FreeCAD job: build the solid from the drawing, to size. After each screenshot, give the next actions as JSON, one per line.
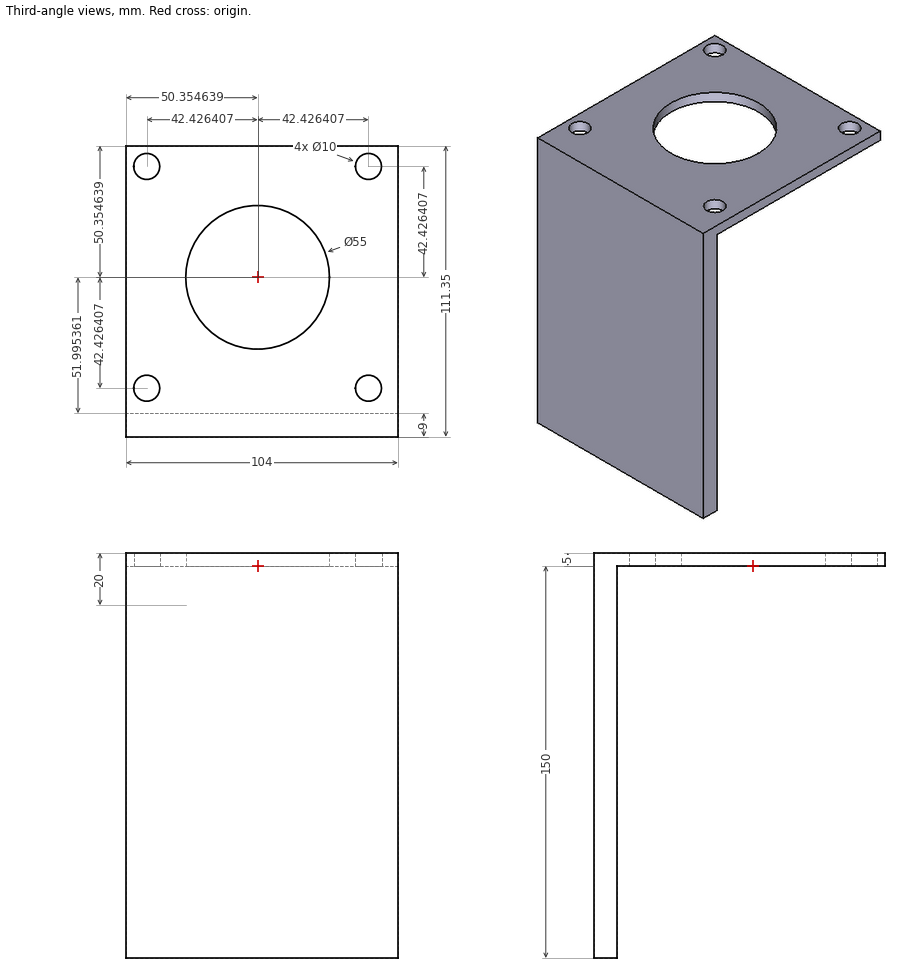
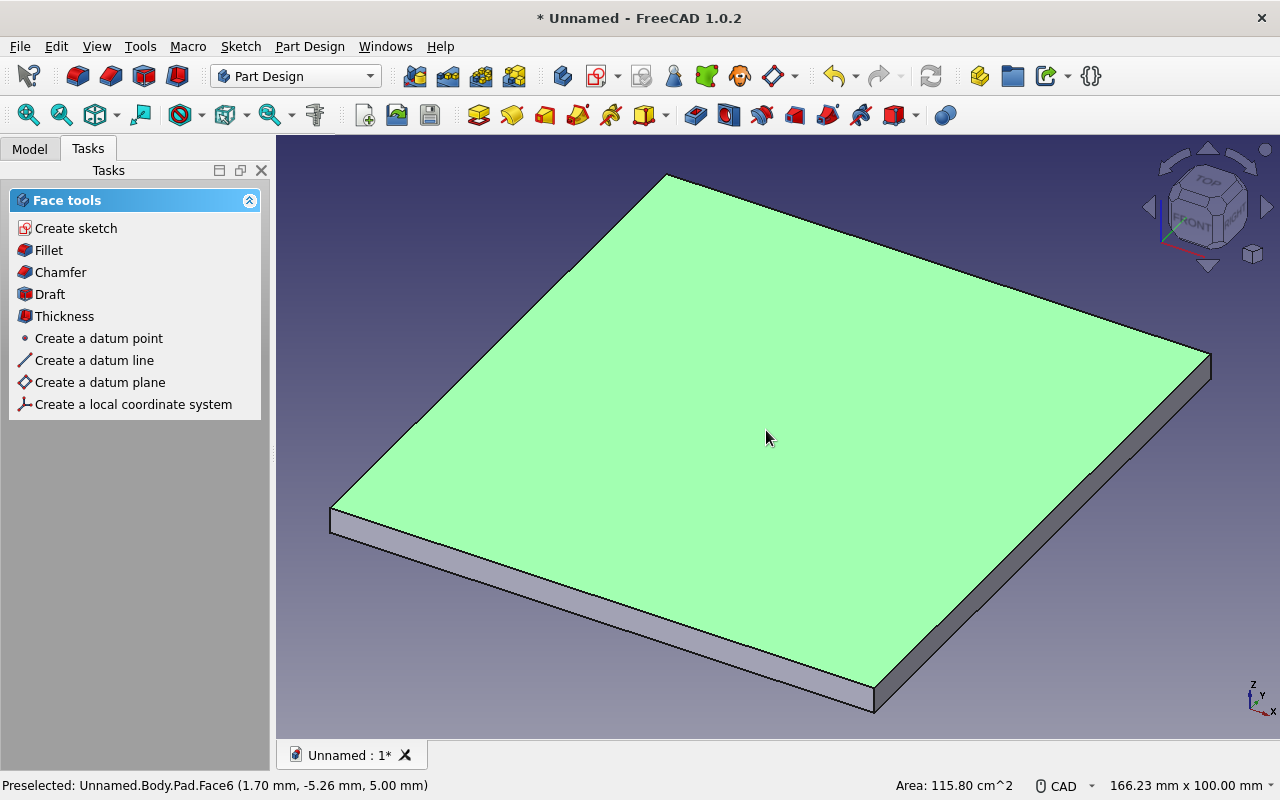
{"action": "left_click", "coordinate": [596, 76]}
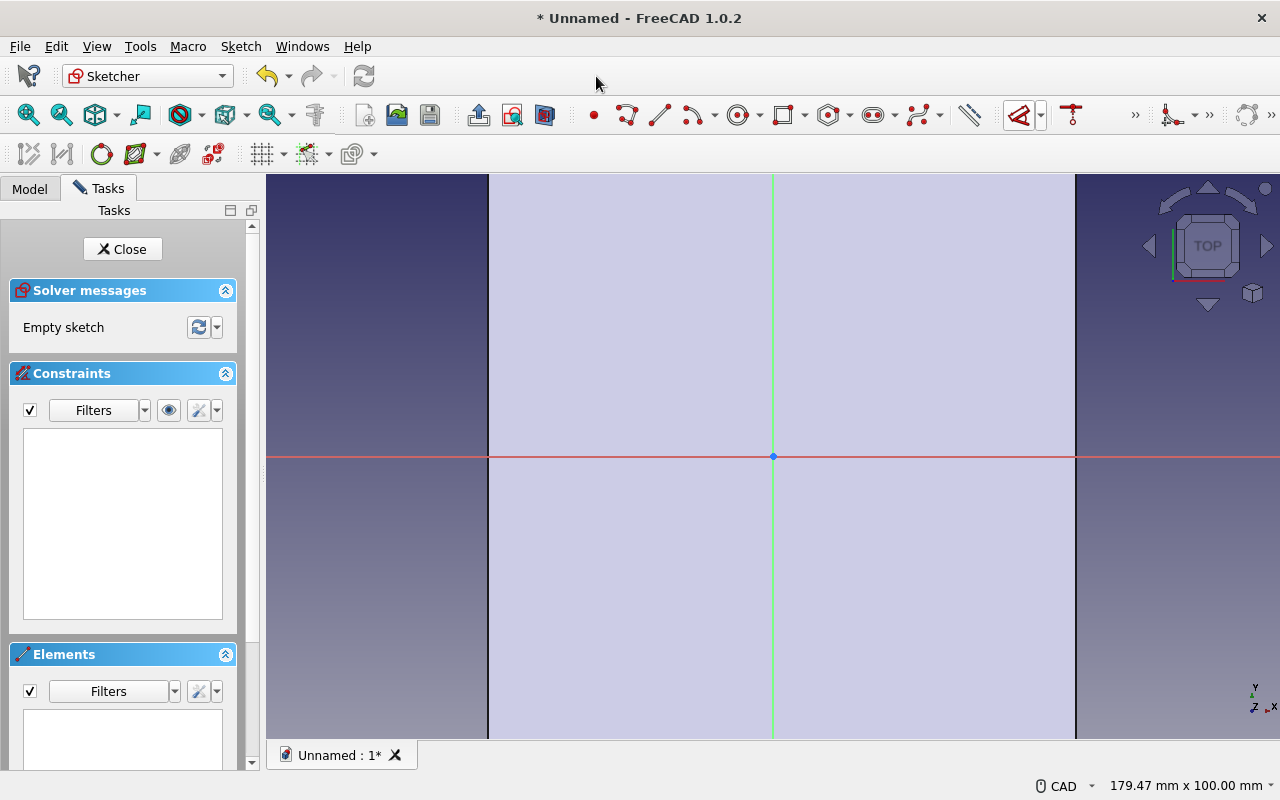
{"action": "key", "text": "g c"}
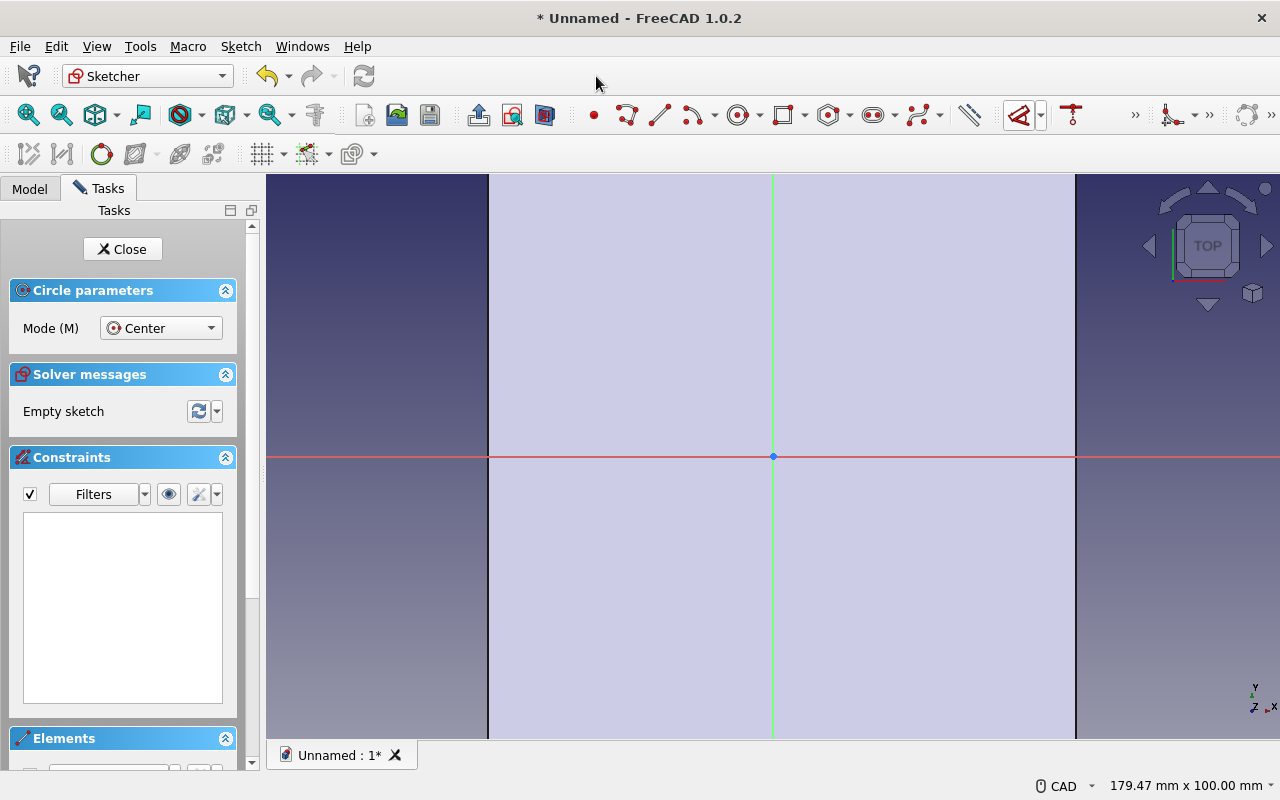
{"action": "left_click", "coordinate": [773, 456]}
{"action": "mouse_move", "coordinate": [883, 347]}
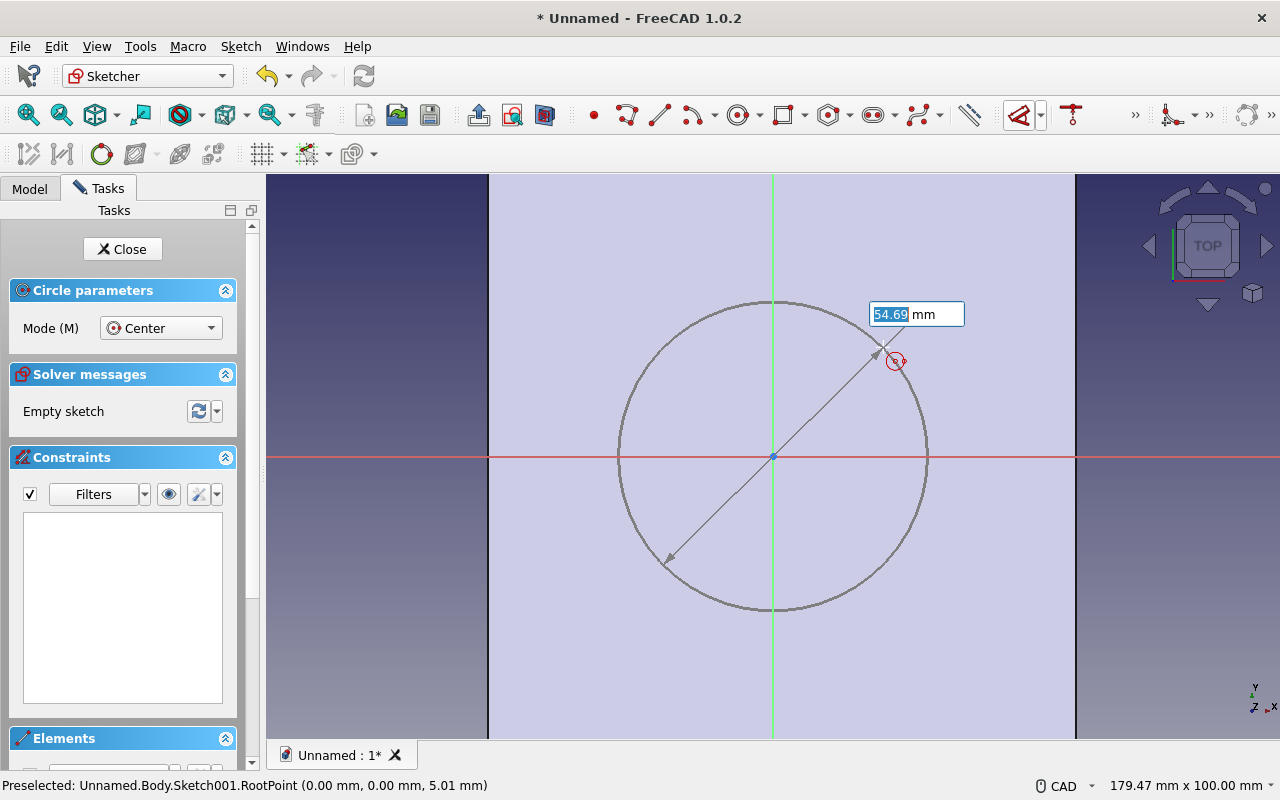
{"action": "type", "text": "55"}
{"action": "key", "text": "Return"}
{"action": "key", "text": "Escape"}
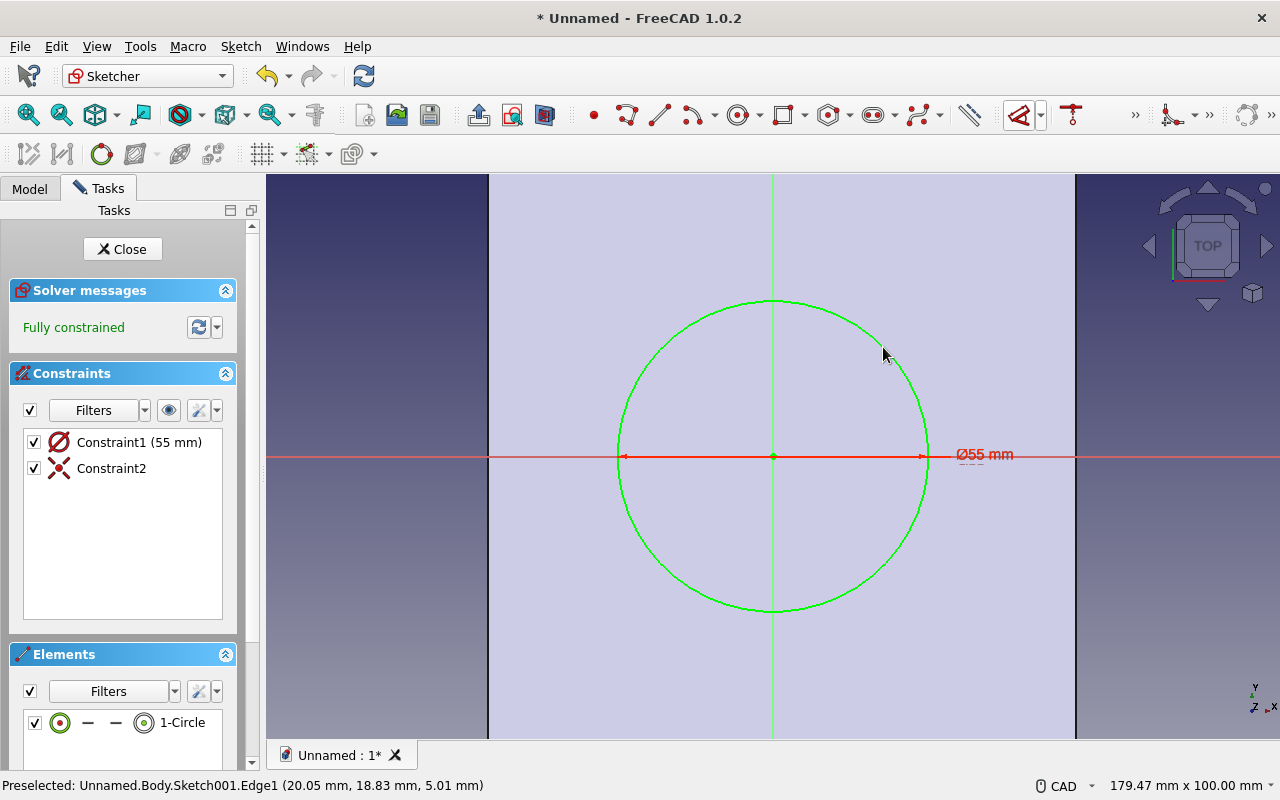
{"action": "left_click", "coordinate": [123, 249]}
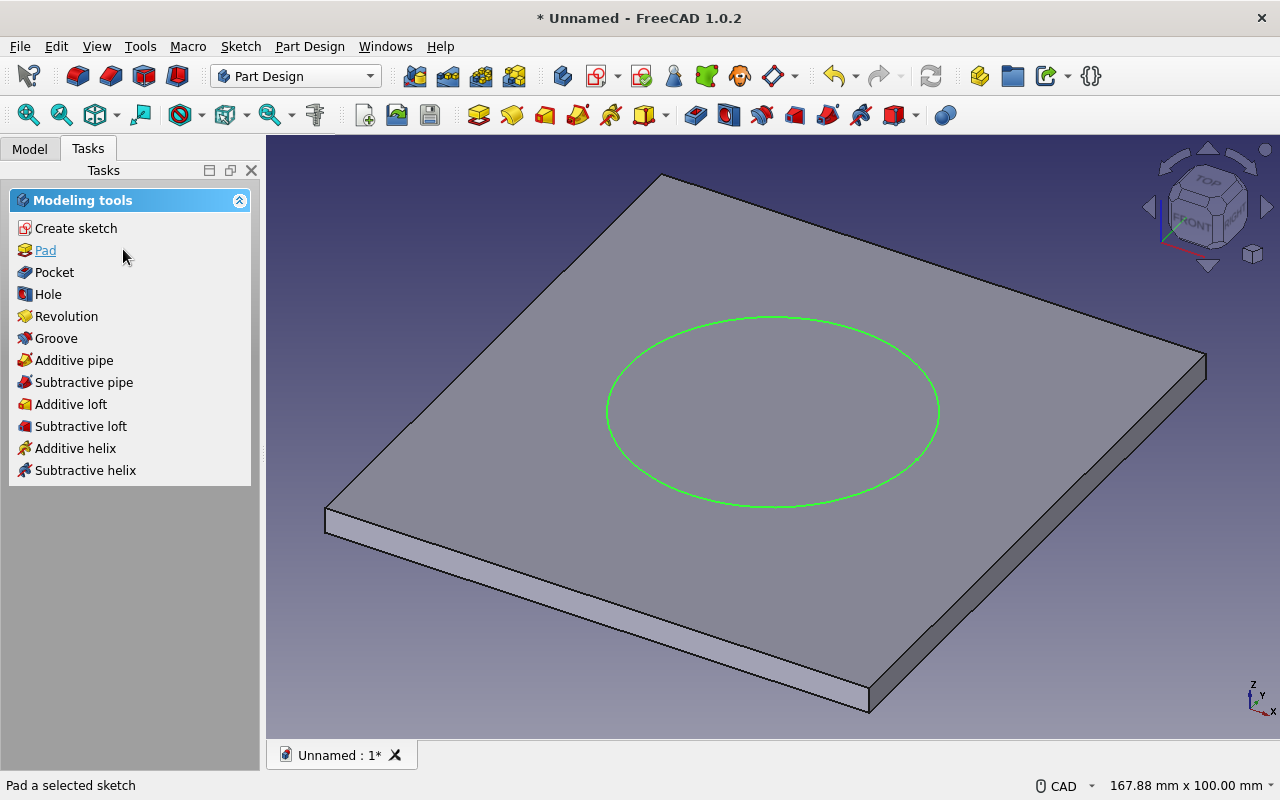
{"action": "left_click", "coordinate": [696, 116]}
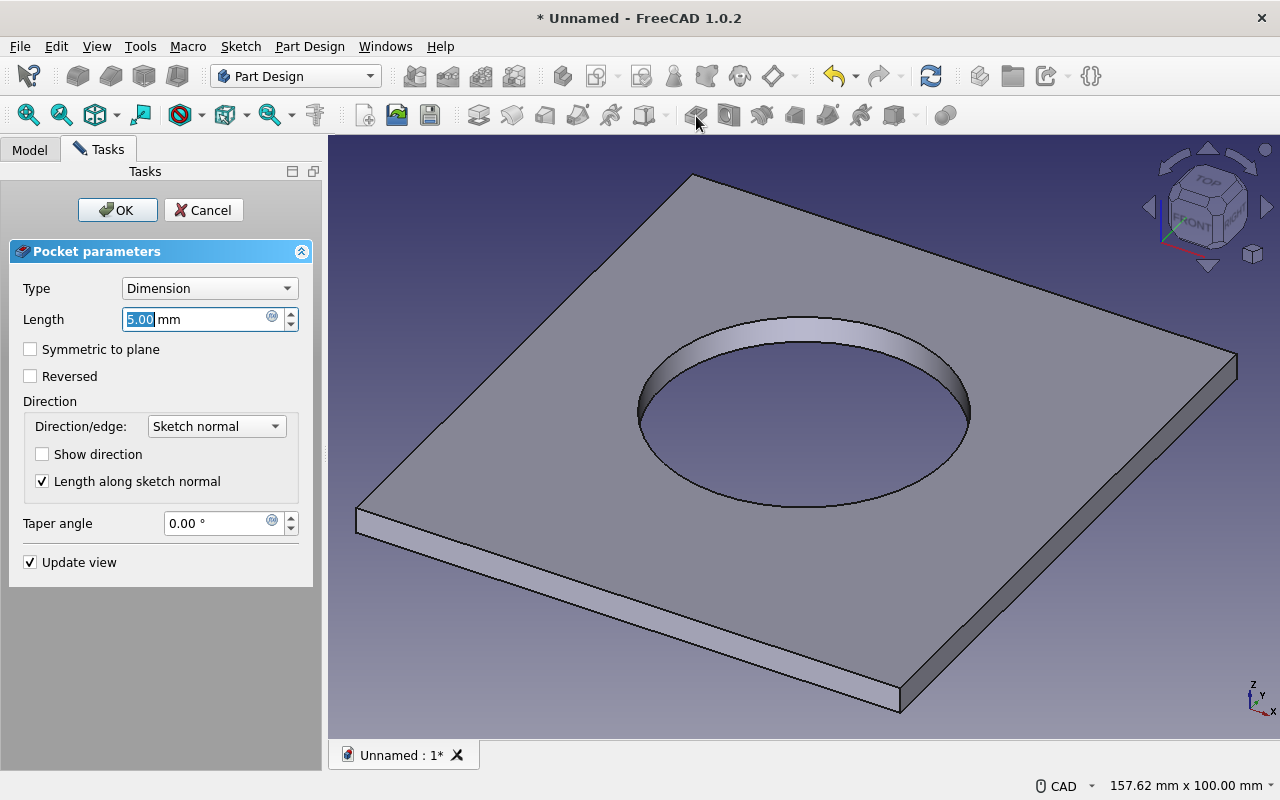
{"action": "type", "text": "20"}
{"action": "key", "text": "Tab"}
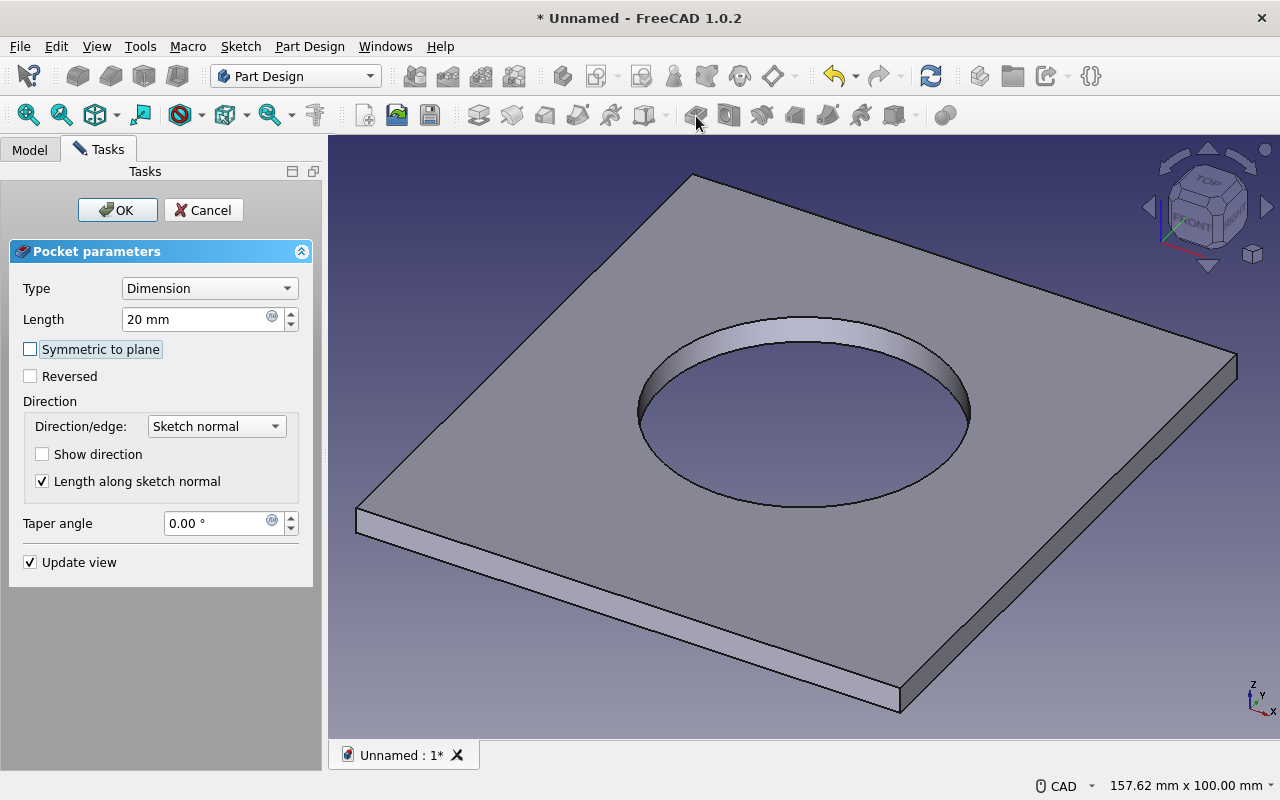
{"action": "left_click", "coordinate": [118, 210]}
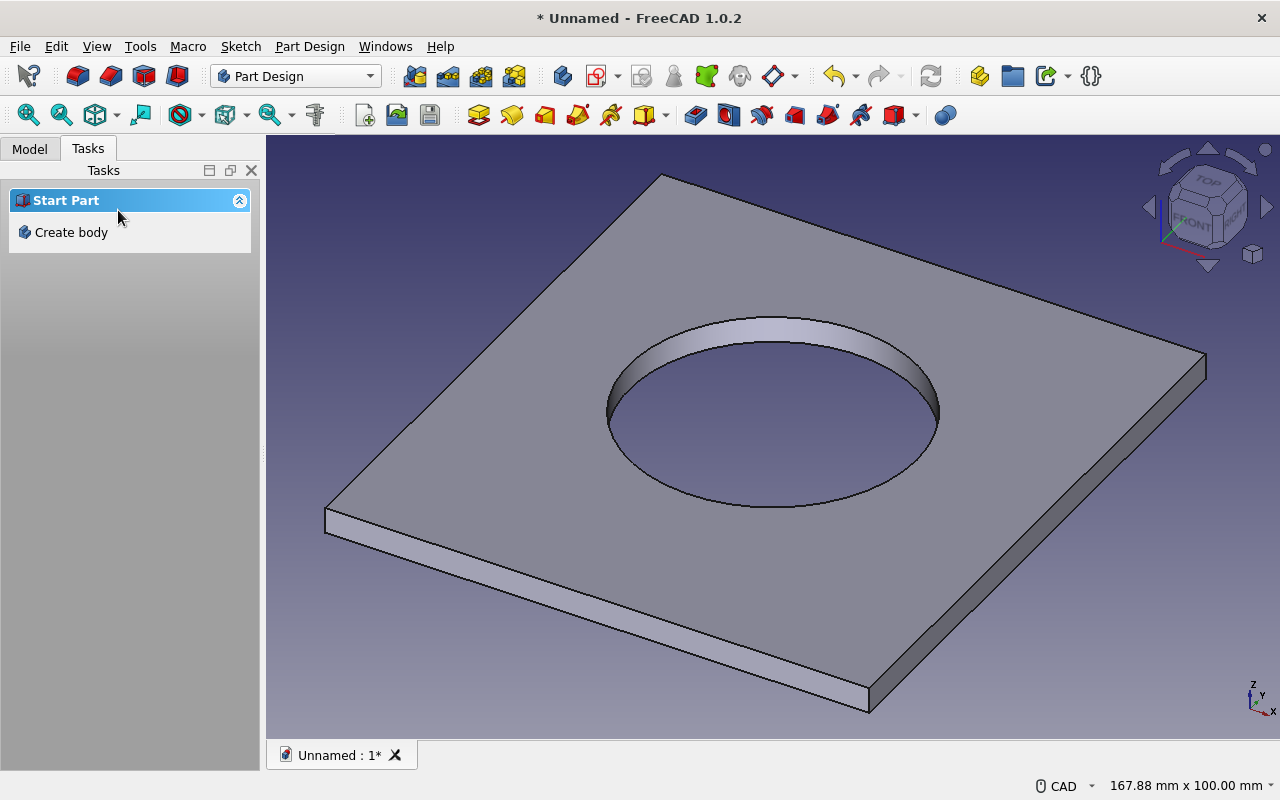
{"action": "left_click", "coordinate": [596, 76]}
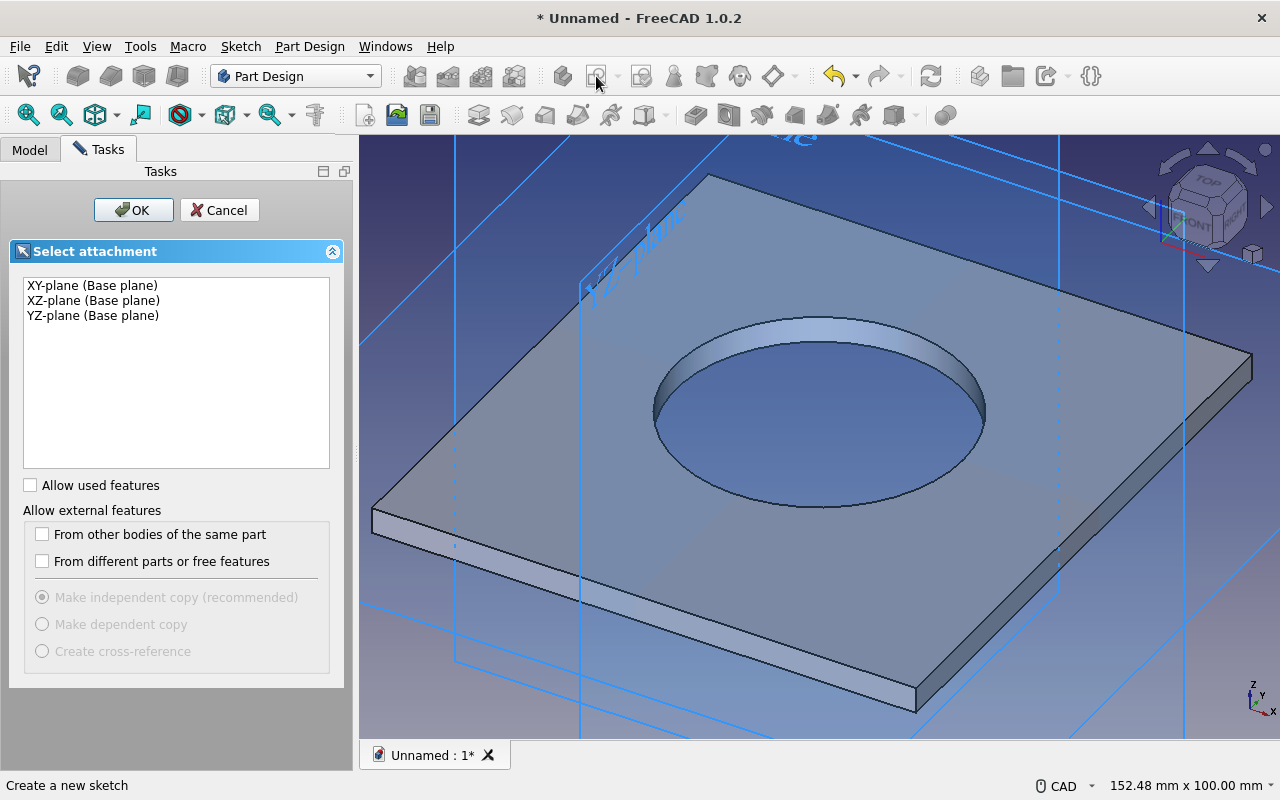
{"action": "left_click", "coordinate": [84, 286]}